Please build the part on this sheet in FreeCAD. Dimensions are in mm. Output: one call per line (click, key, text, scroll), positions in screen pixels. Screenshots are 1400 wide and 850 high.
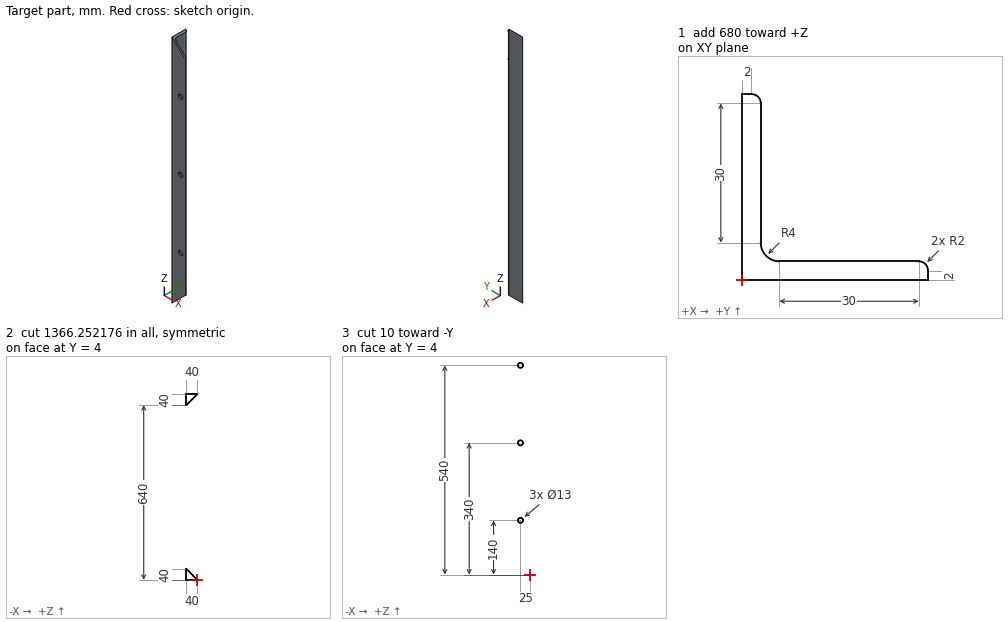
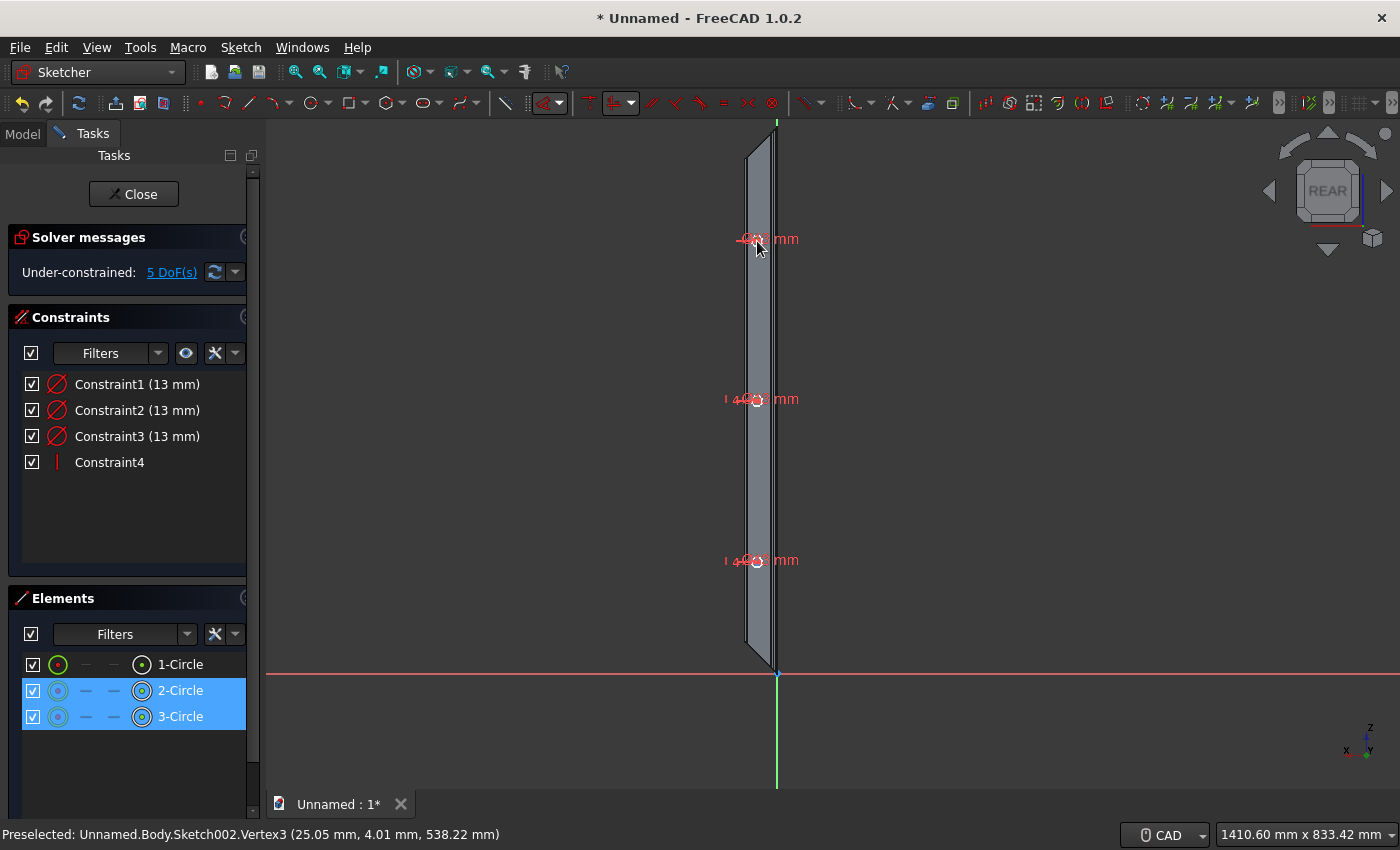
click(634, 104)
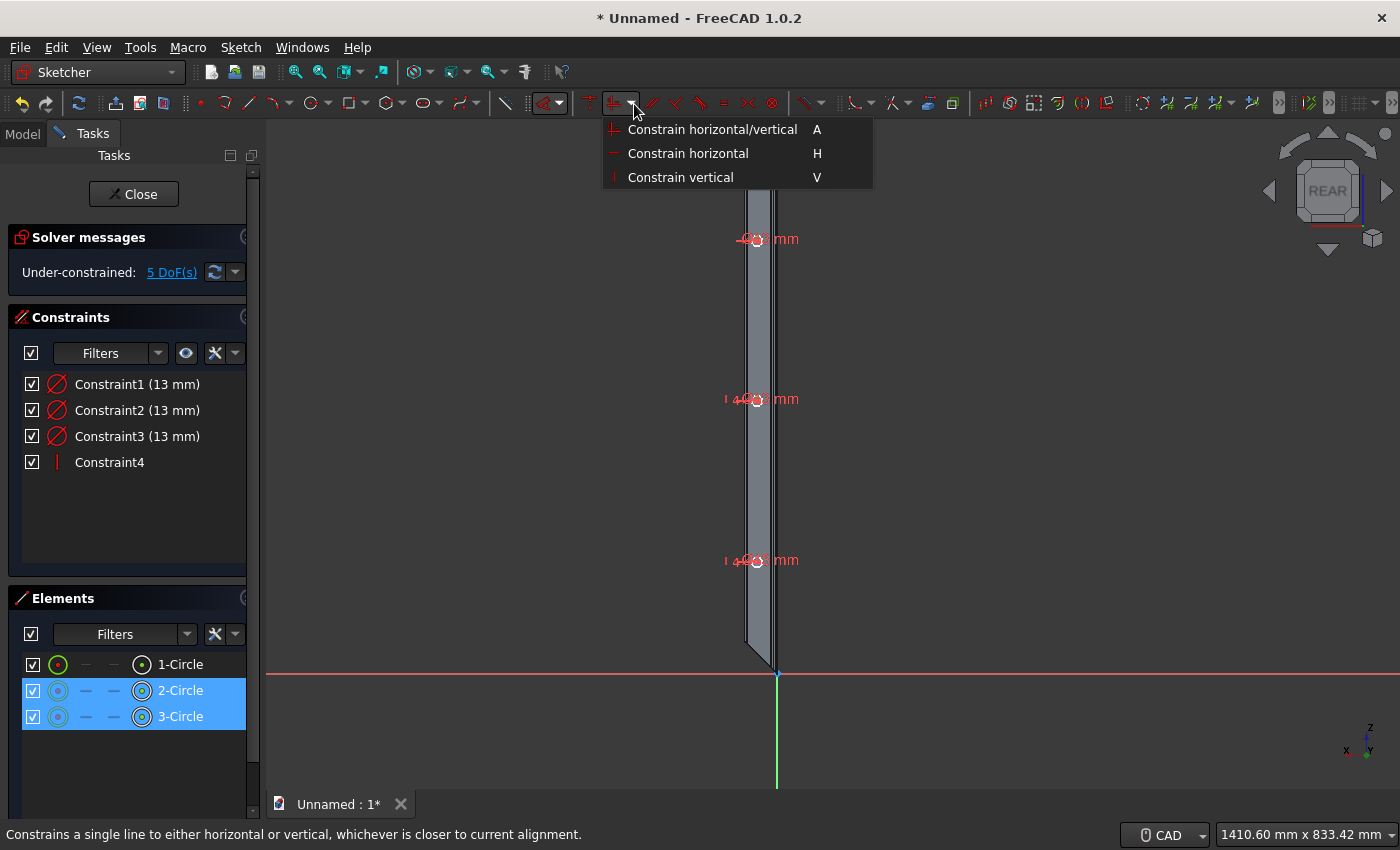
click(738, 177)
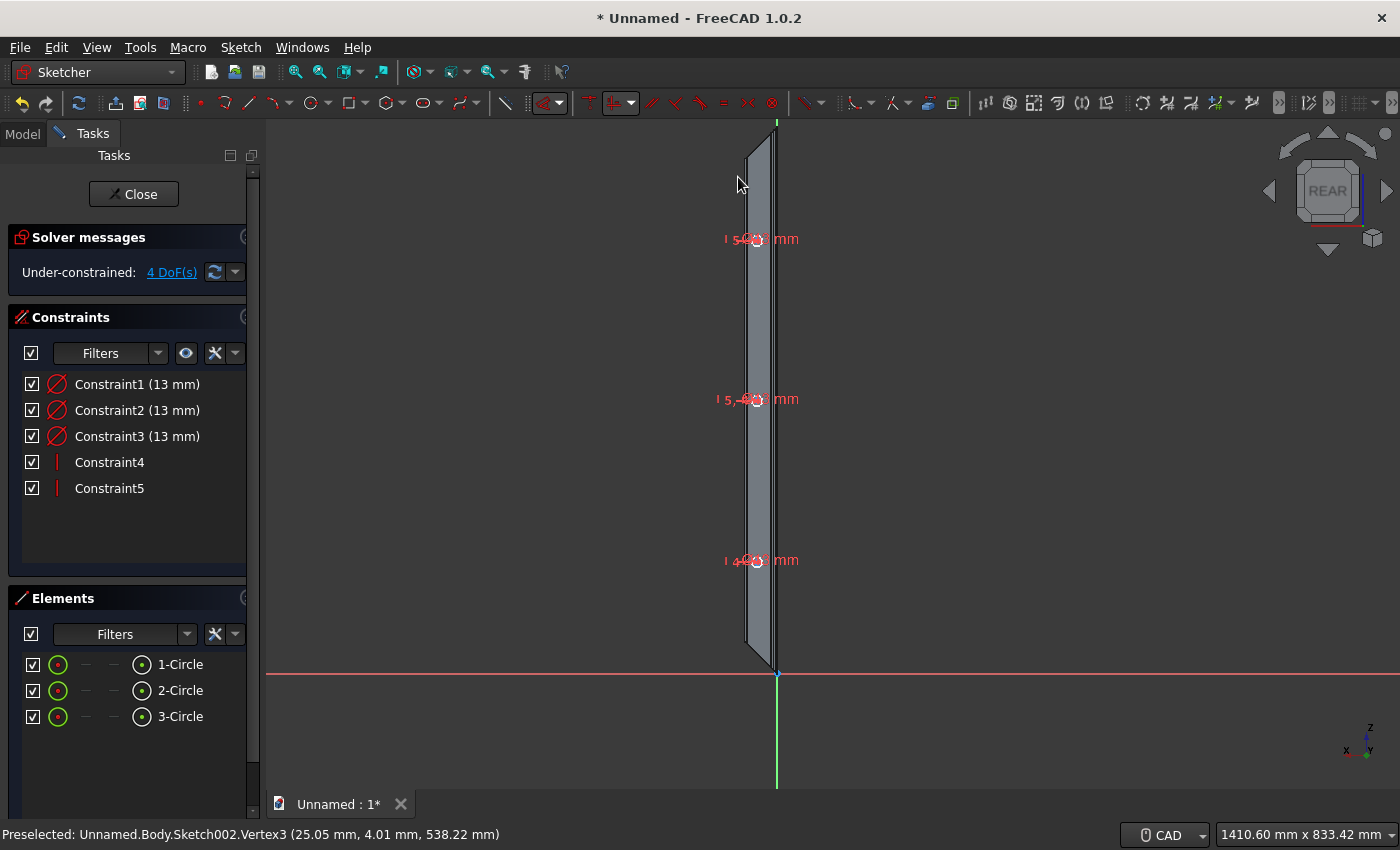
scroll(757, 562, up, 4)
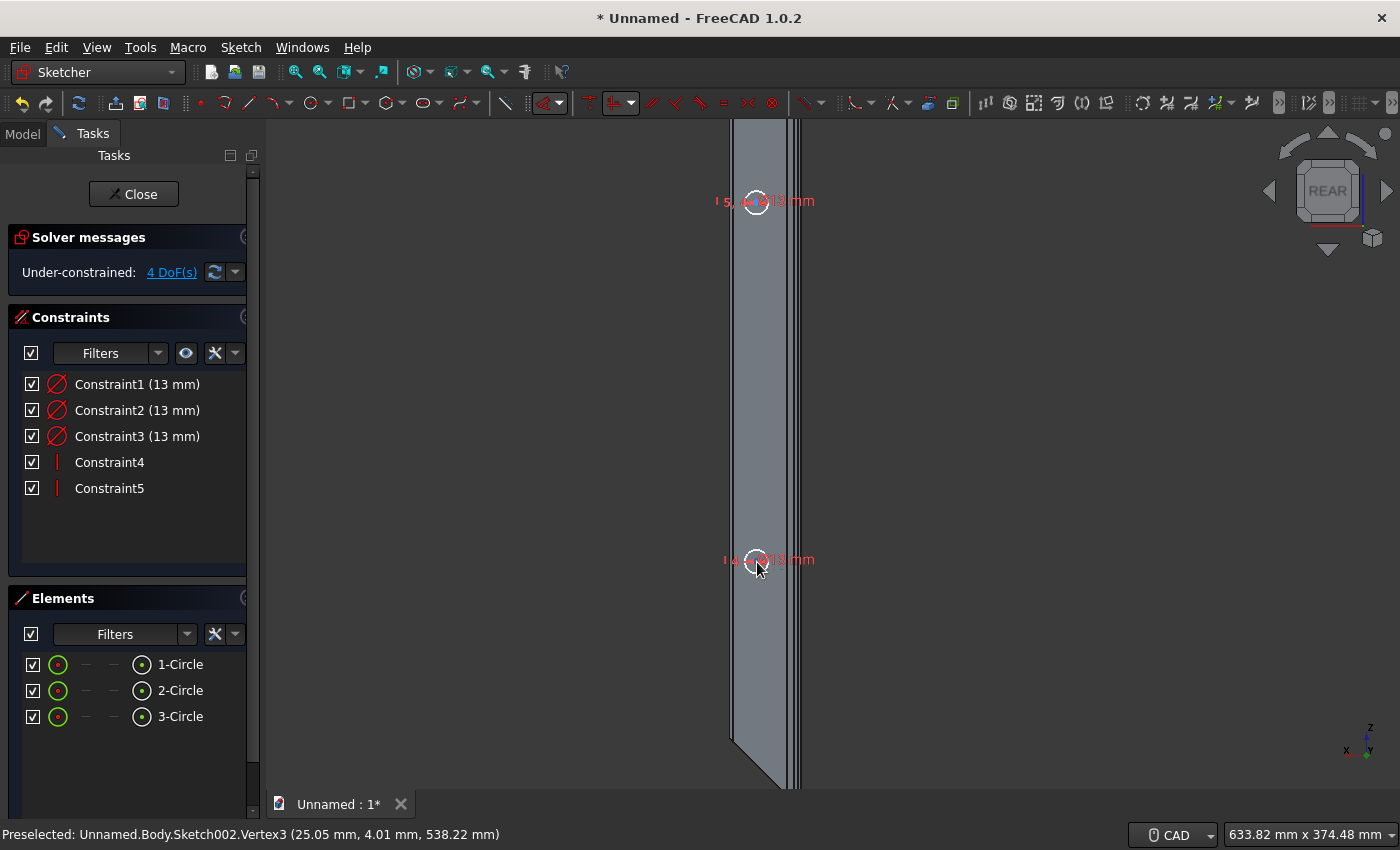
click(756, 562)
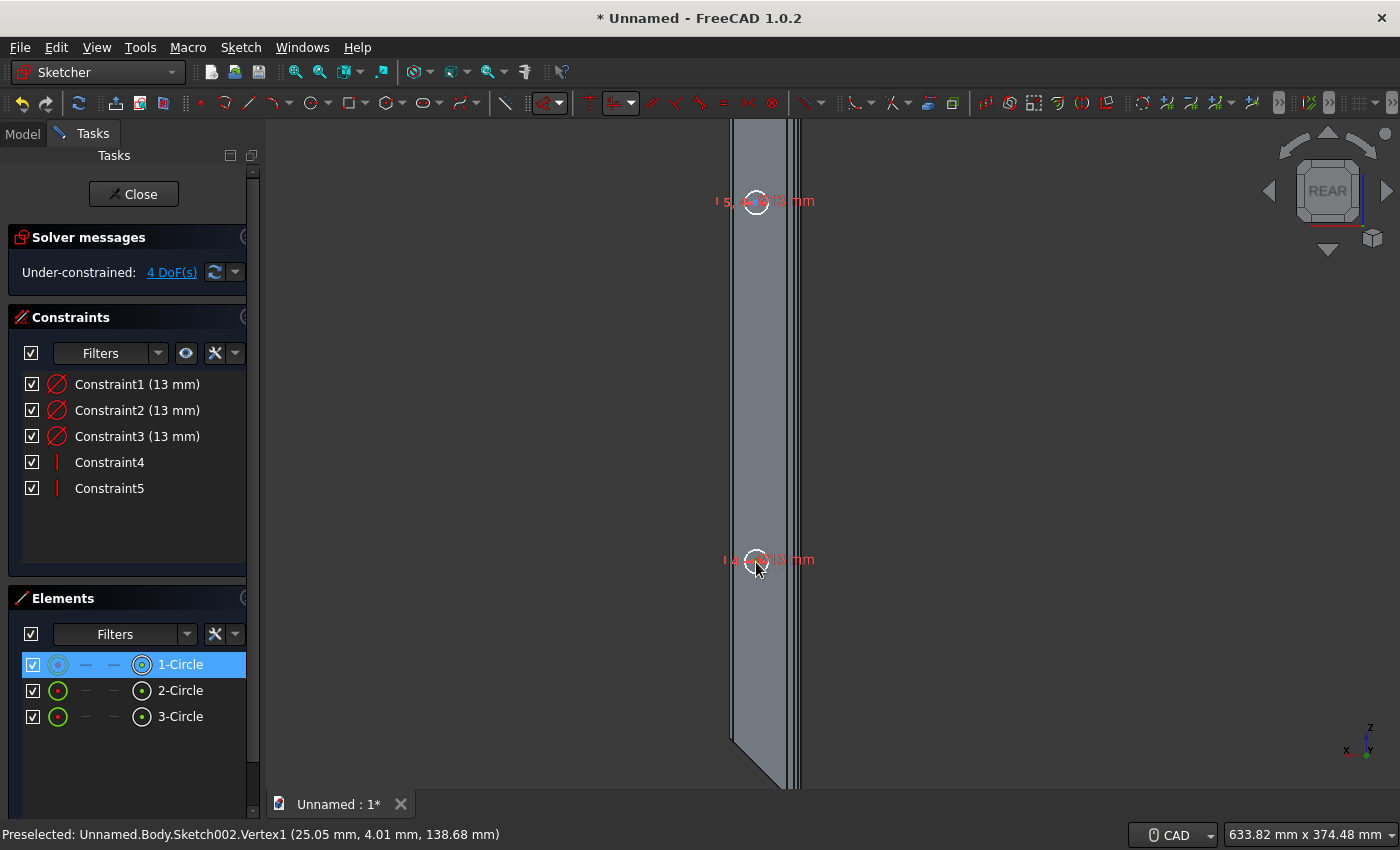
key(l)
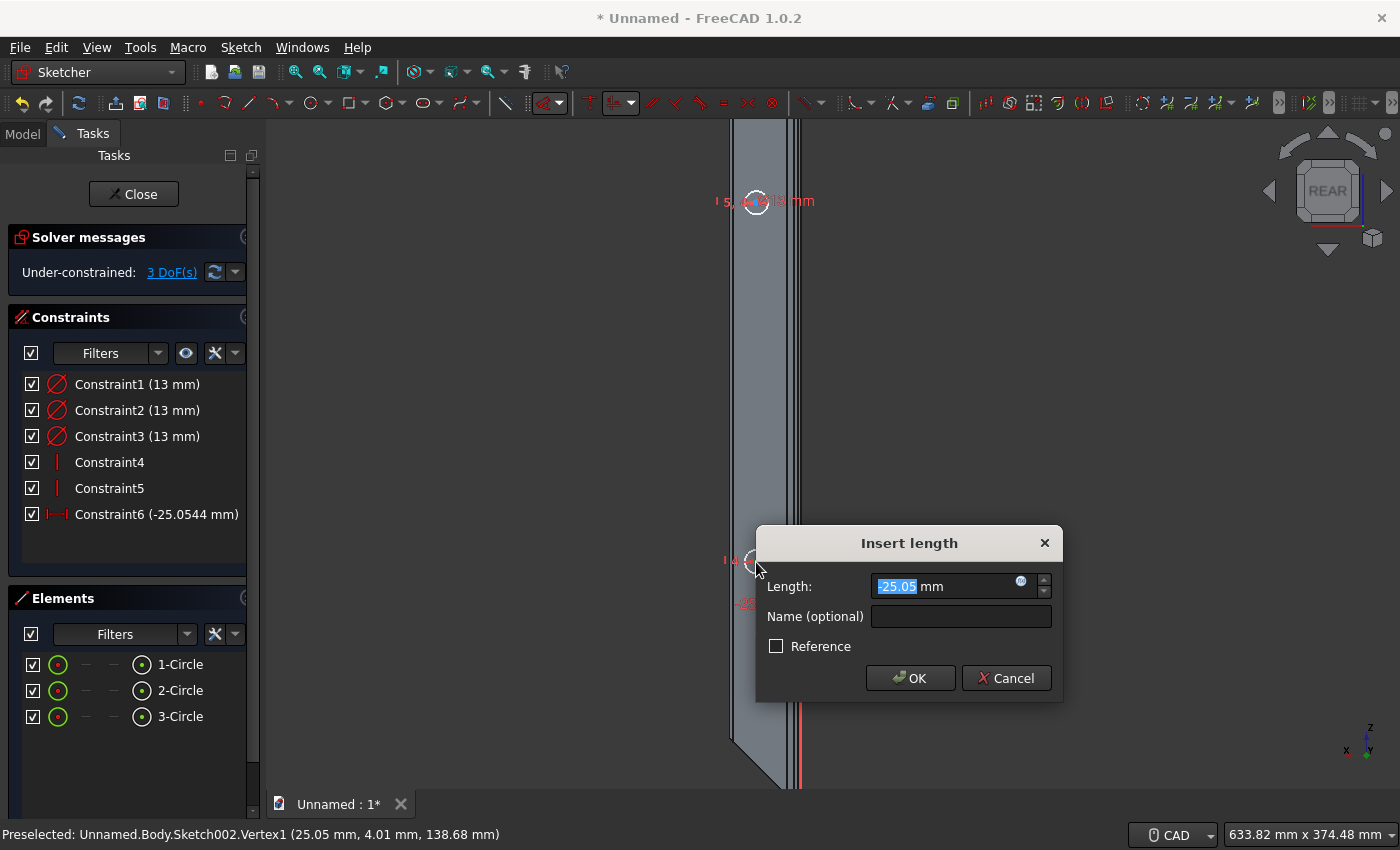
text(-25)
key(Return)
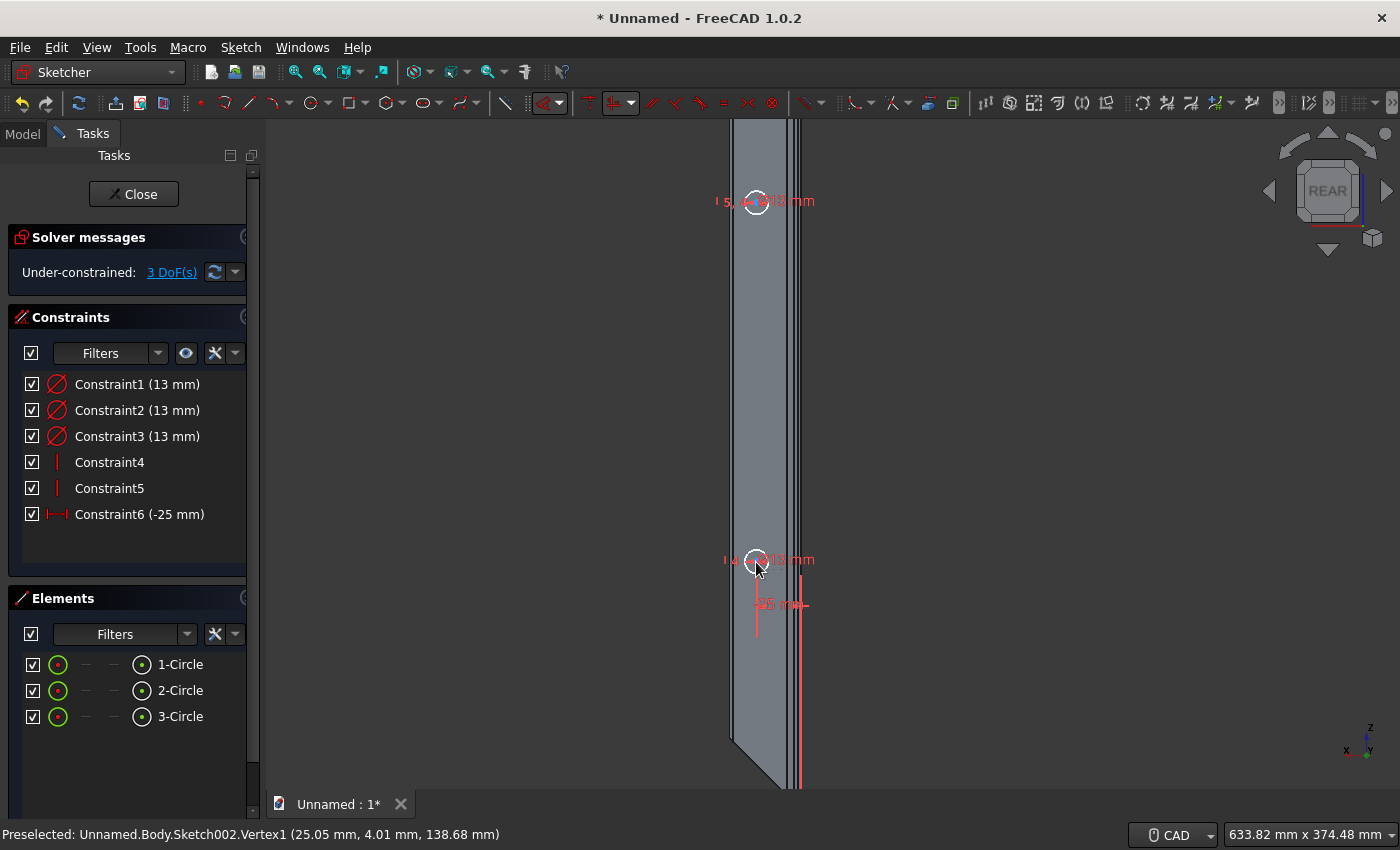
click(757, 562)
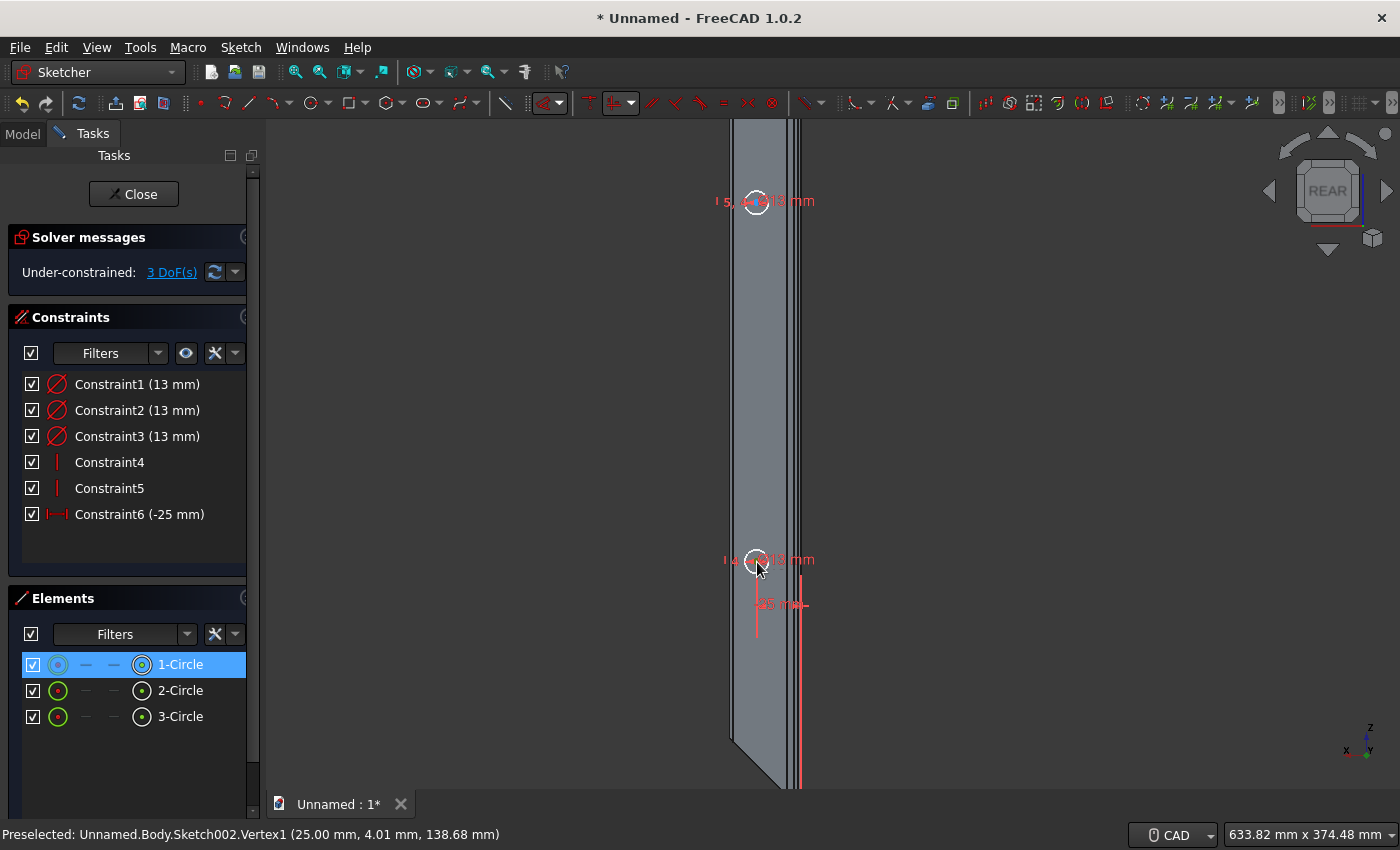
click(562, 104)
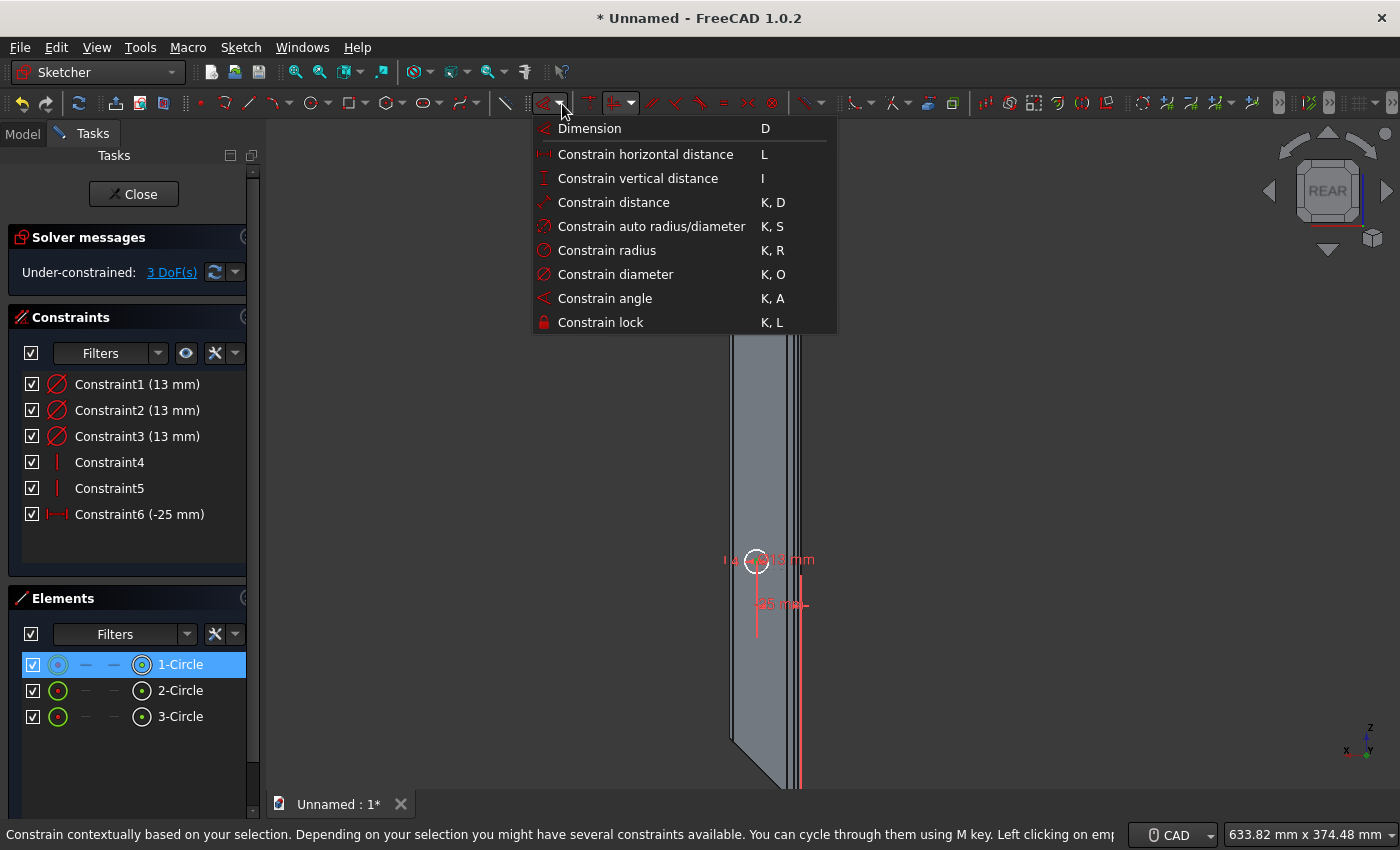
click(685, 178)